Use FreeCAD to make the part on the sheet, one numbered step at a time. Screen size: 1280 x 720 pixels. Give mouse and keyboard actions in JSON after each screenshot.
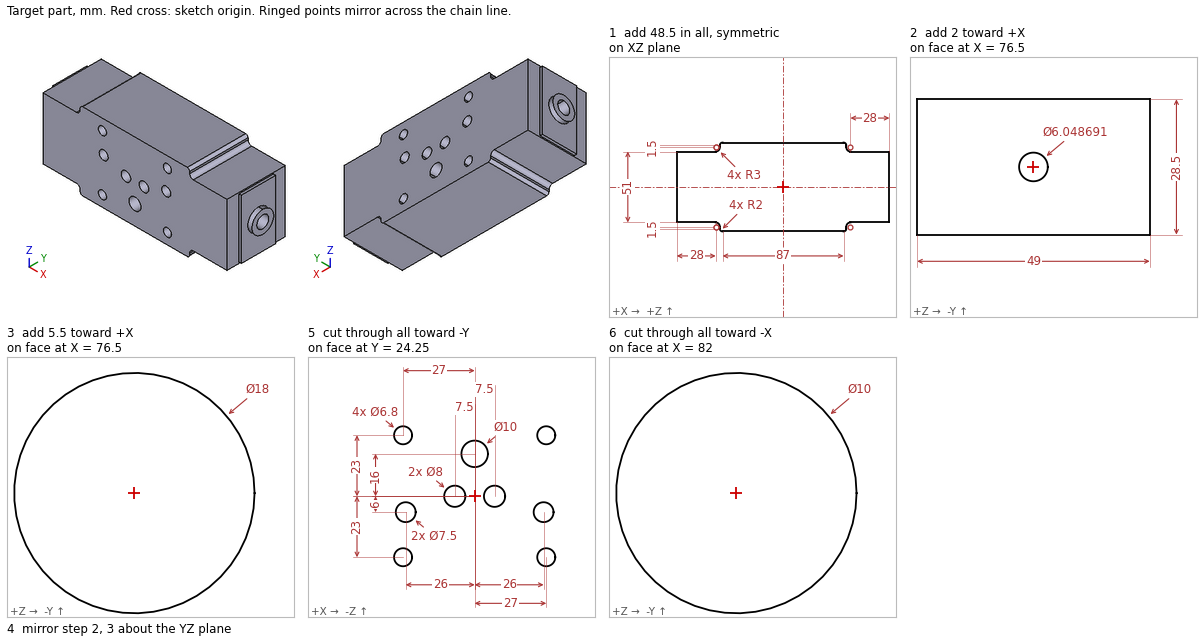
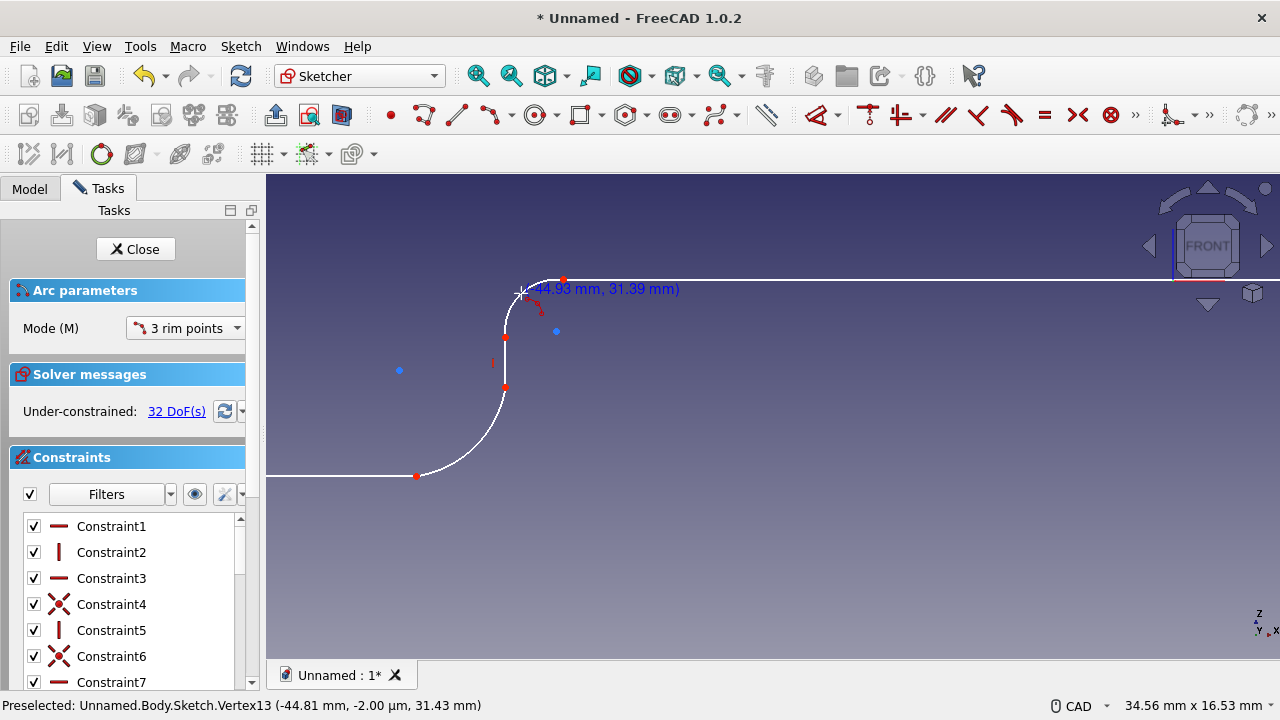
{"action": "scroll", "coordinate": [527, 291], "scroll_direction": "down", "scroll_amount": 10}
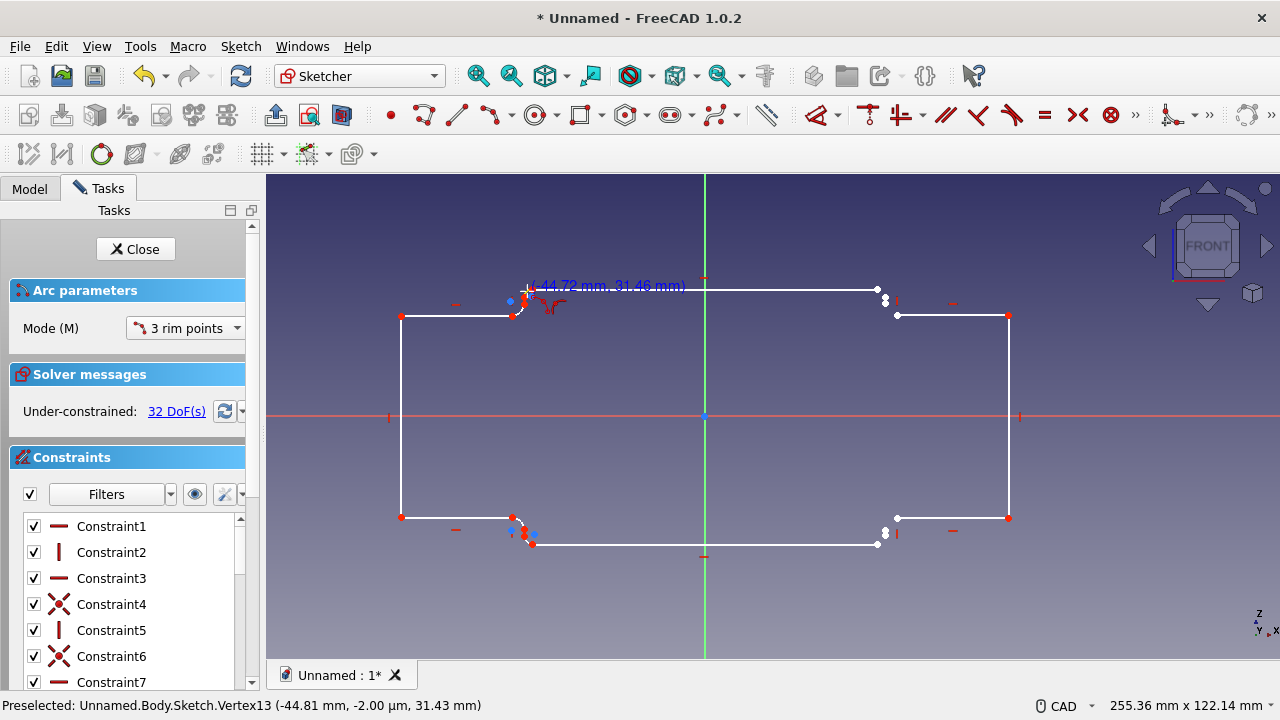
{"action": "scroll", "coordinate": [878, 289], "scroll_direction": "up", "scroll_amount": 2}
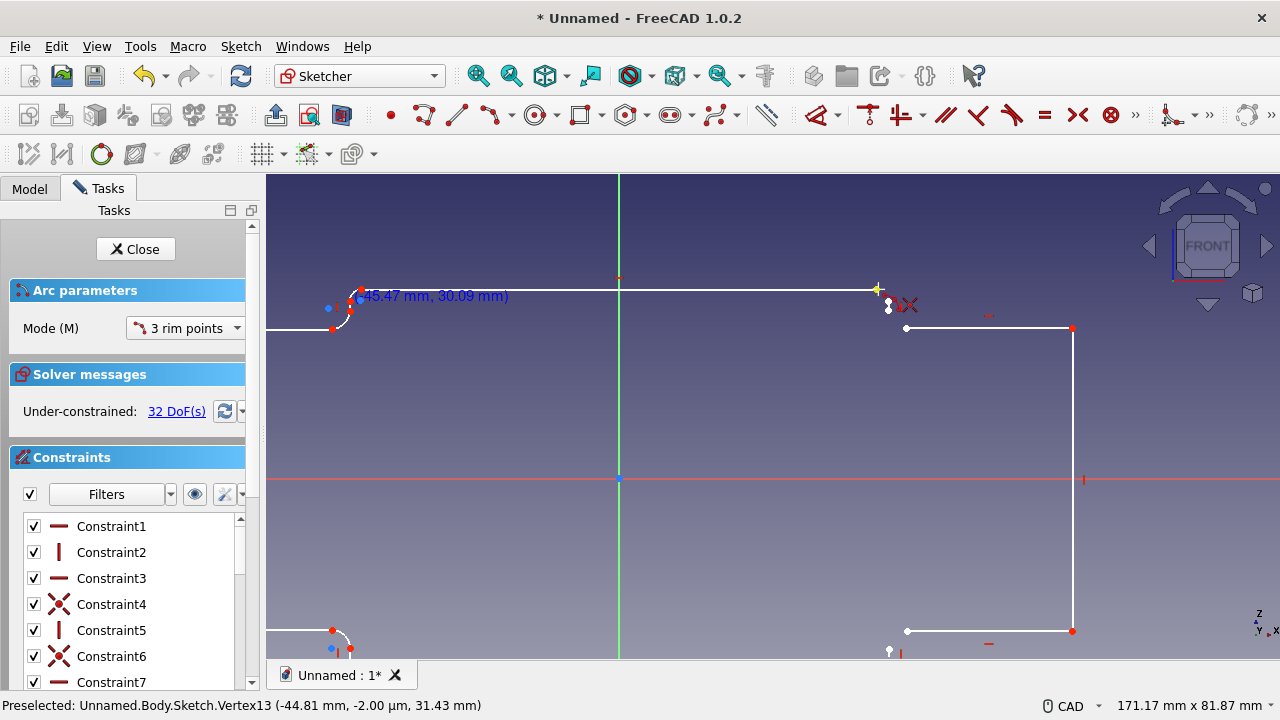
{"action": "left_click", "coordinate": [877, 290]}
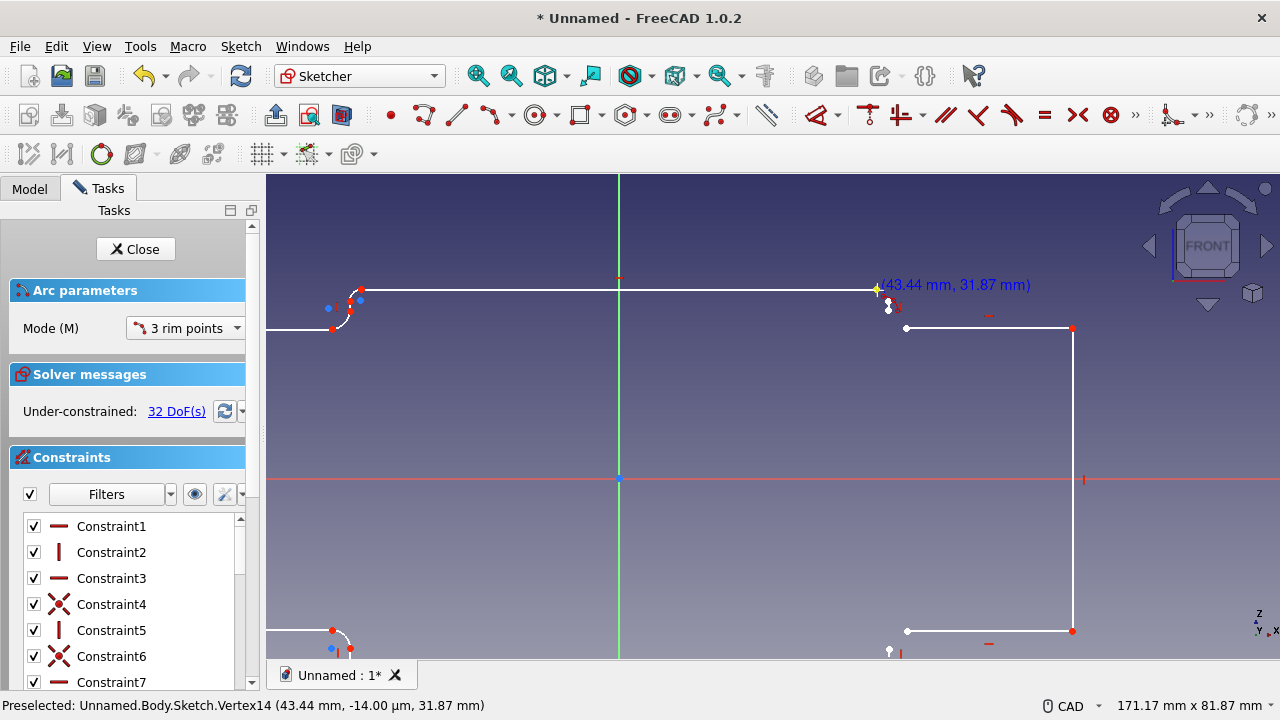
{"action": "scroll", "coordinate": [889, 301], "scroll_direction": "up", "scroll_amount": 7}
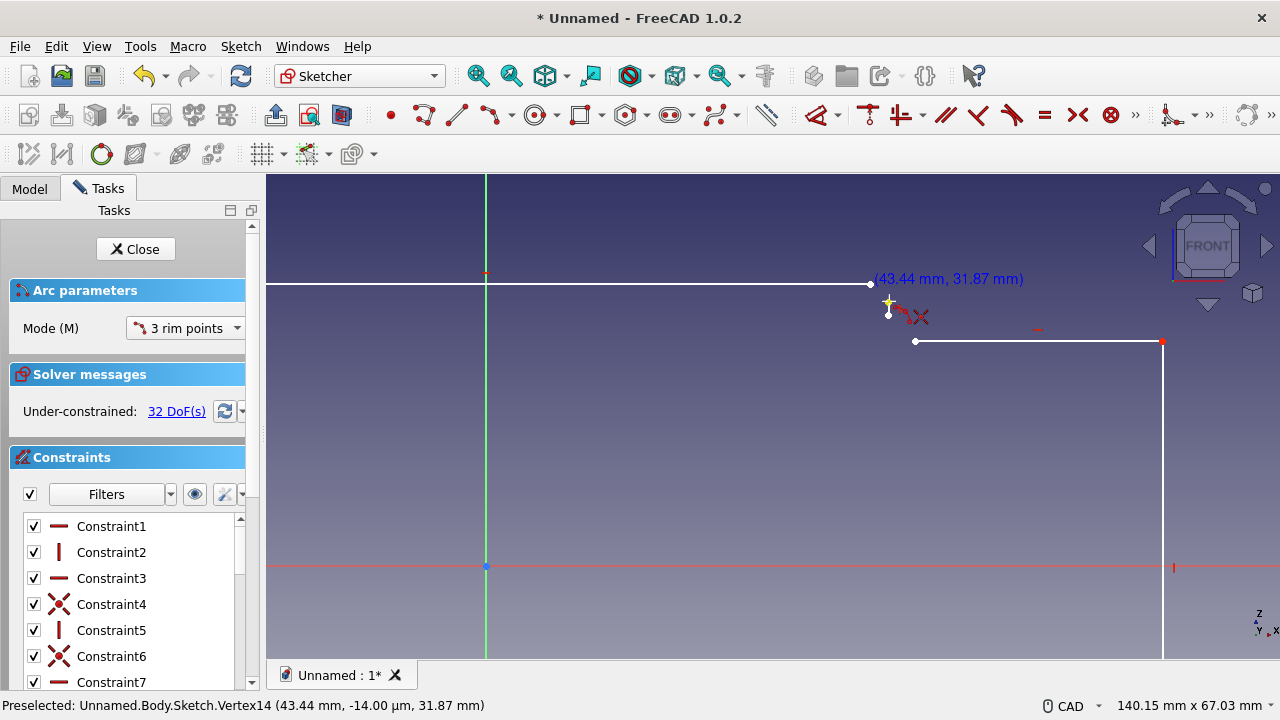
{"action": "left_click", "coordinate": [887, 304]}
{"action": "left_click", "coordinate": [872, 266]}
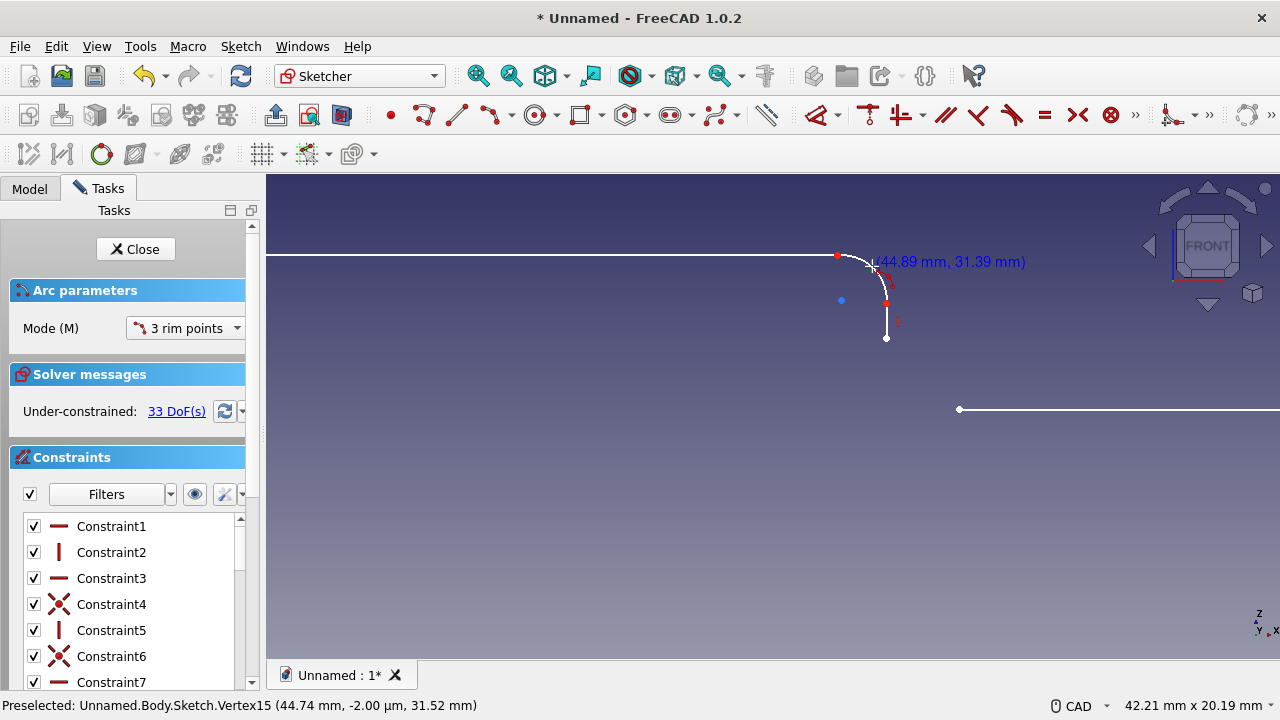
{"action": "left_click", "coordinate": [887, 339]}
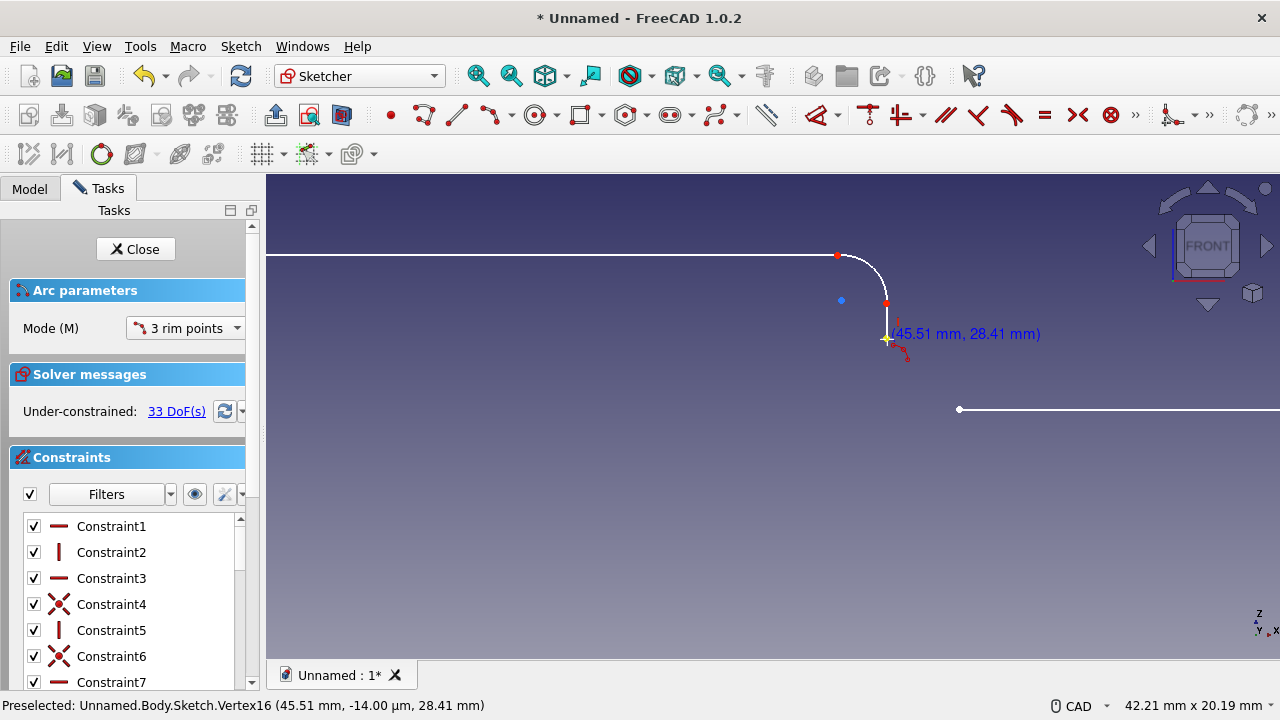
{"action": "scroll", "coordinate": [885, 297], "scroll_direction": "down", "scroll_amount": 9}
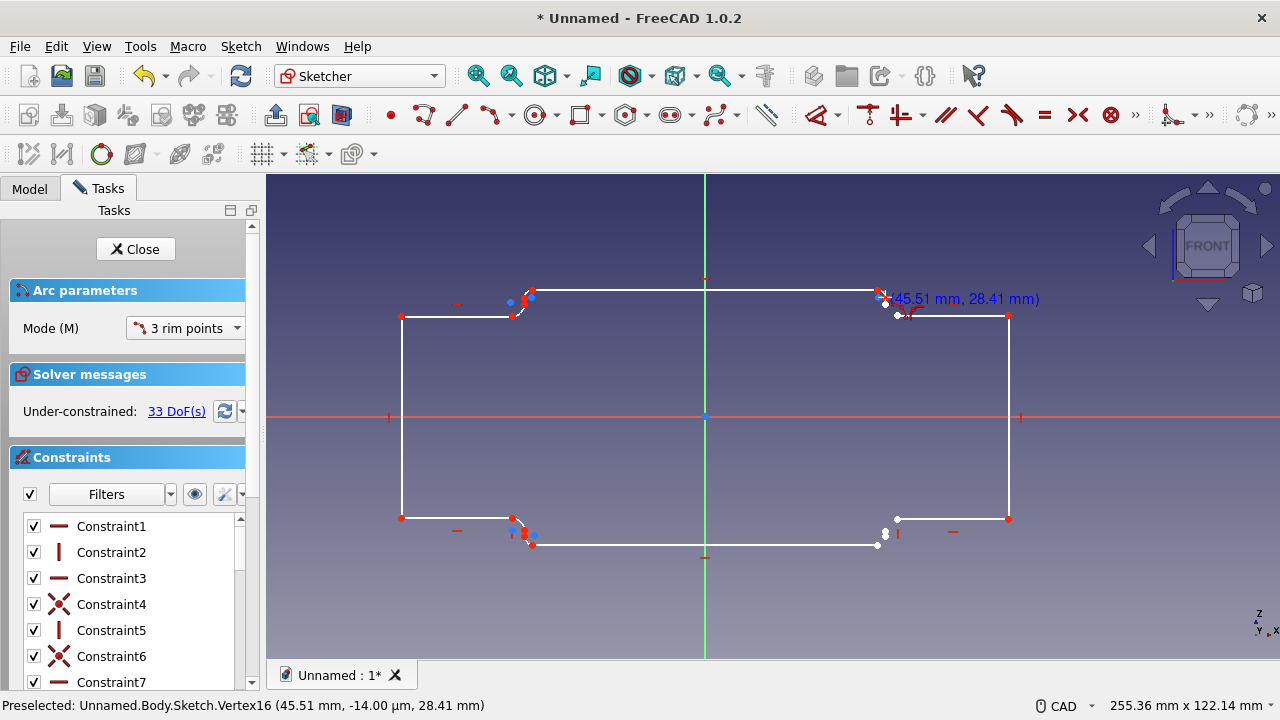
{"action": "left_click", "coordinate": [898, 316]}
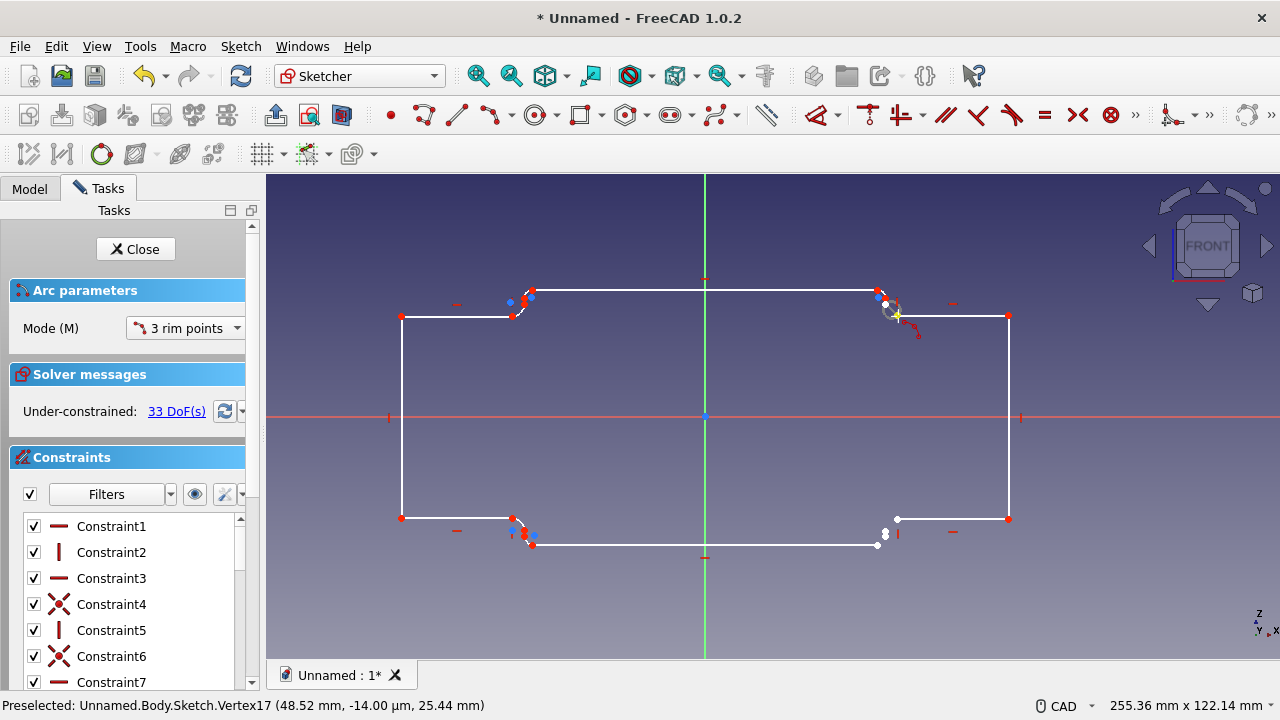
{"action": "scroll", "coordinate": [889, 312], "scroll_direction": "up", "scroll_amount": 8}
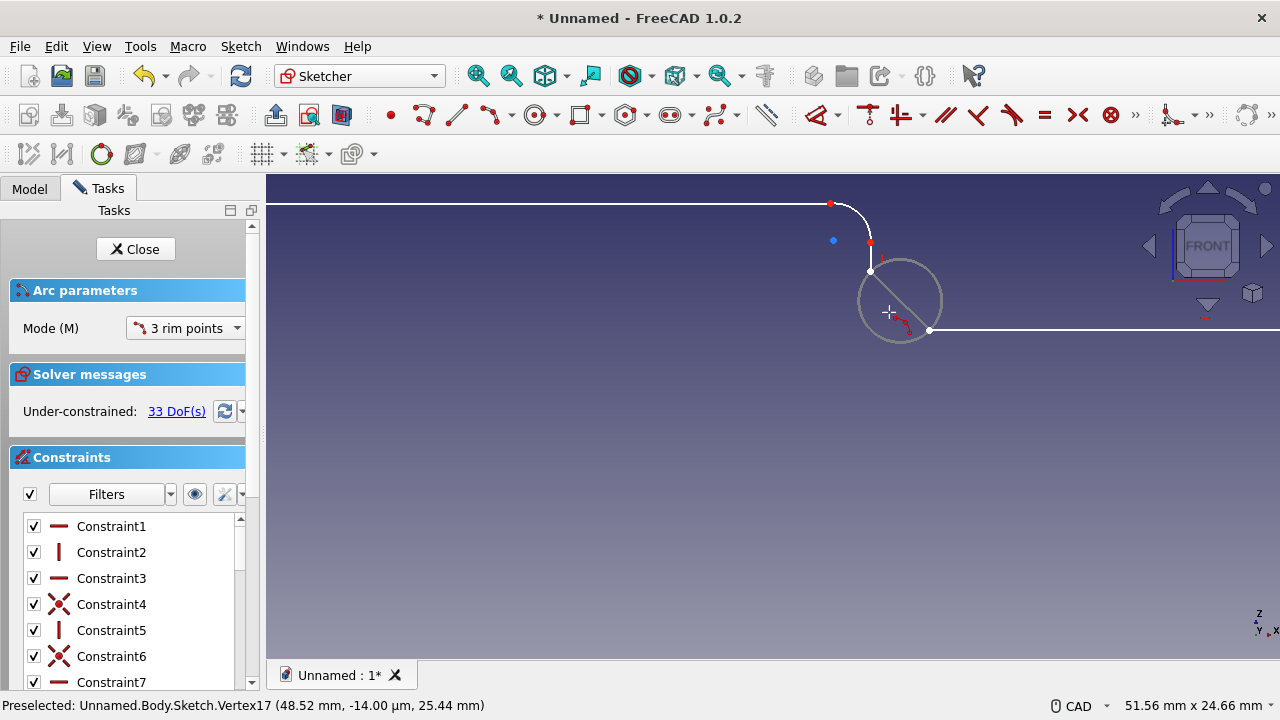
{"action": "left_click", "coordinate": [888, 312]}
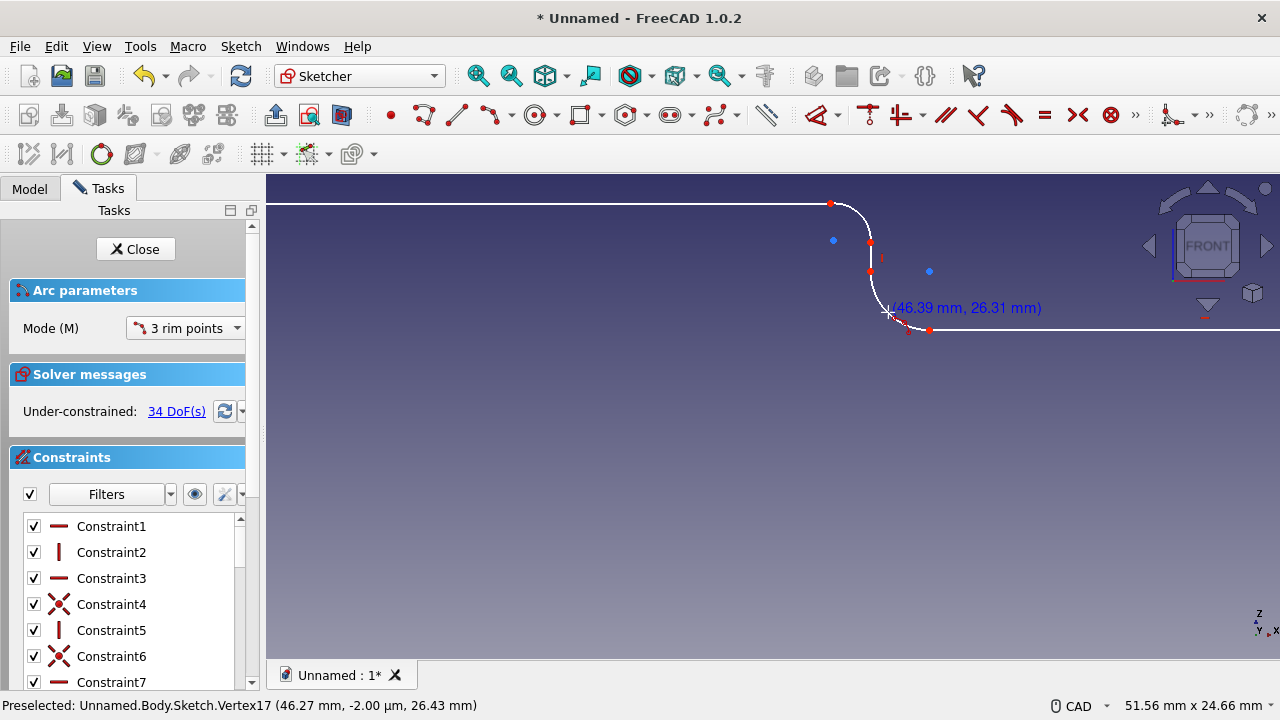
{"action": "scroll", "coordinate": [889, 312], "scroll_direction": "down", "scroll_amount": 8}